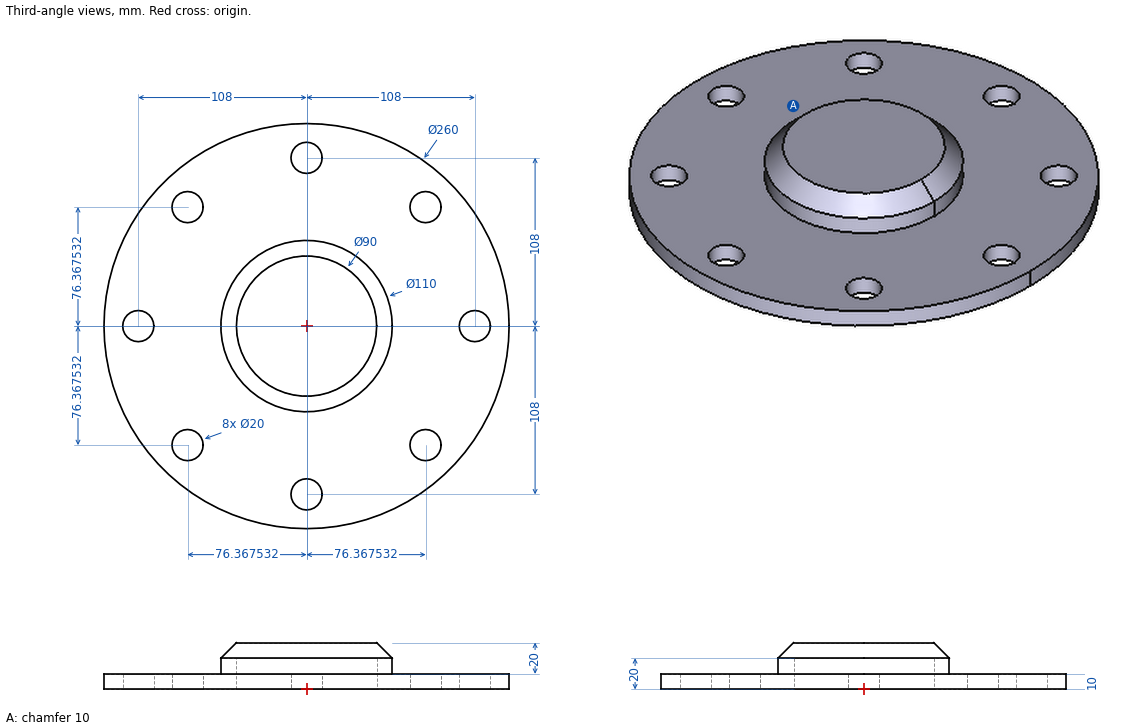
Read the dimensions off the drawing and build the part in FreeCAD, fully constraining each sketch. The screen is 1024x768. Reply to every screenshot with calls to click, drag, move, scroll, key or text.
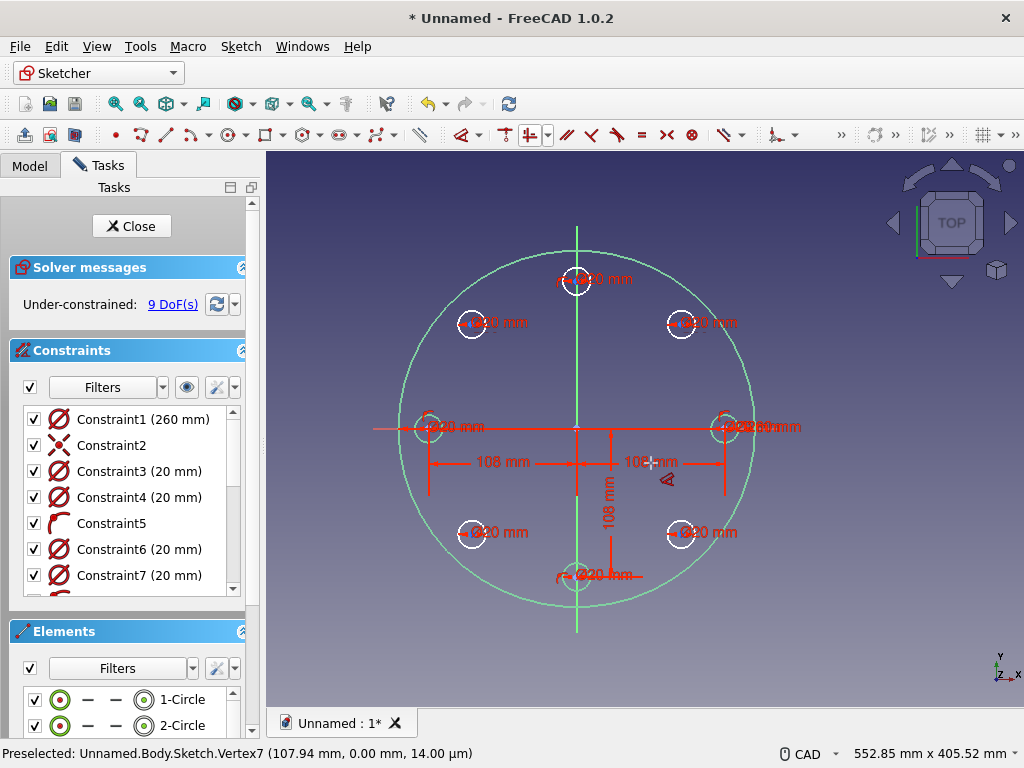
click(577, 281)
click(611, 355)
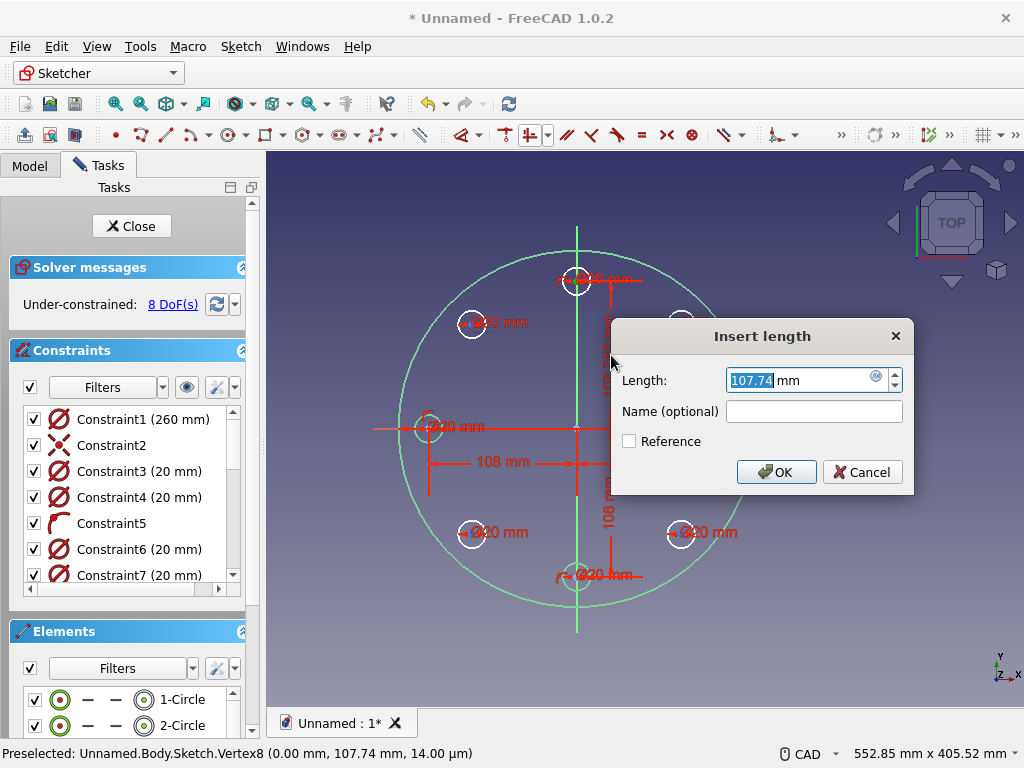
text(108)
key(Return)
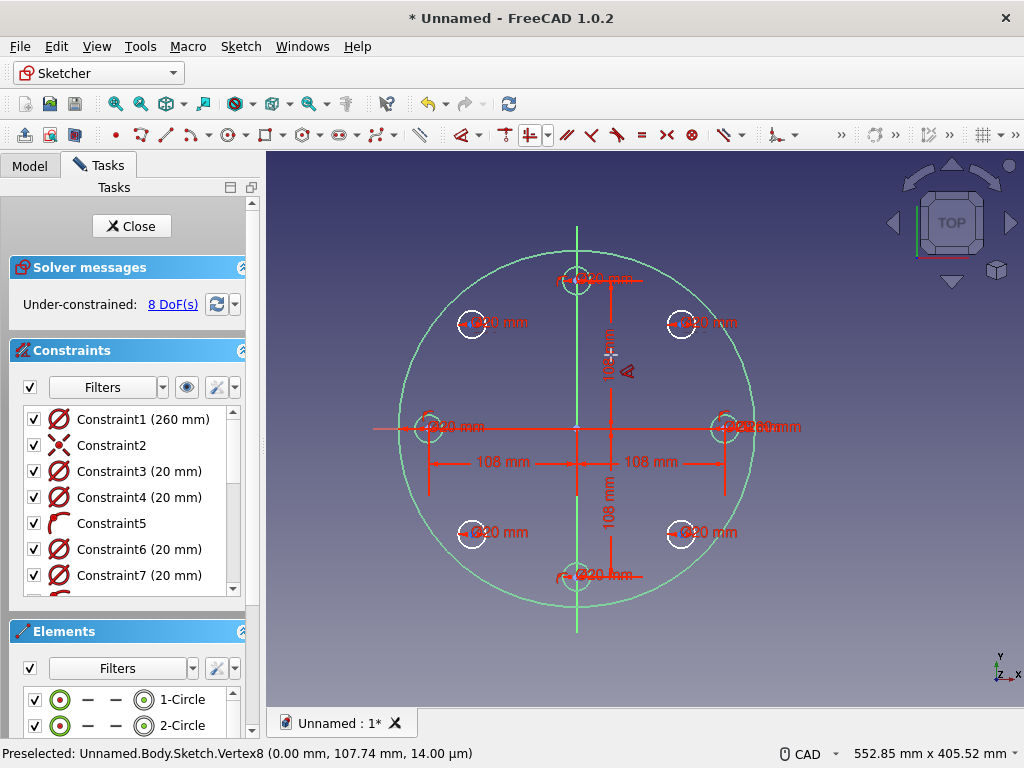
click(472, 534)
click(524, 568)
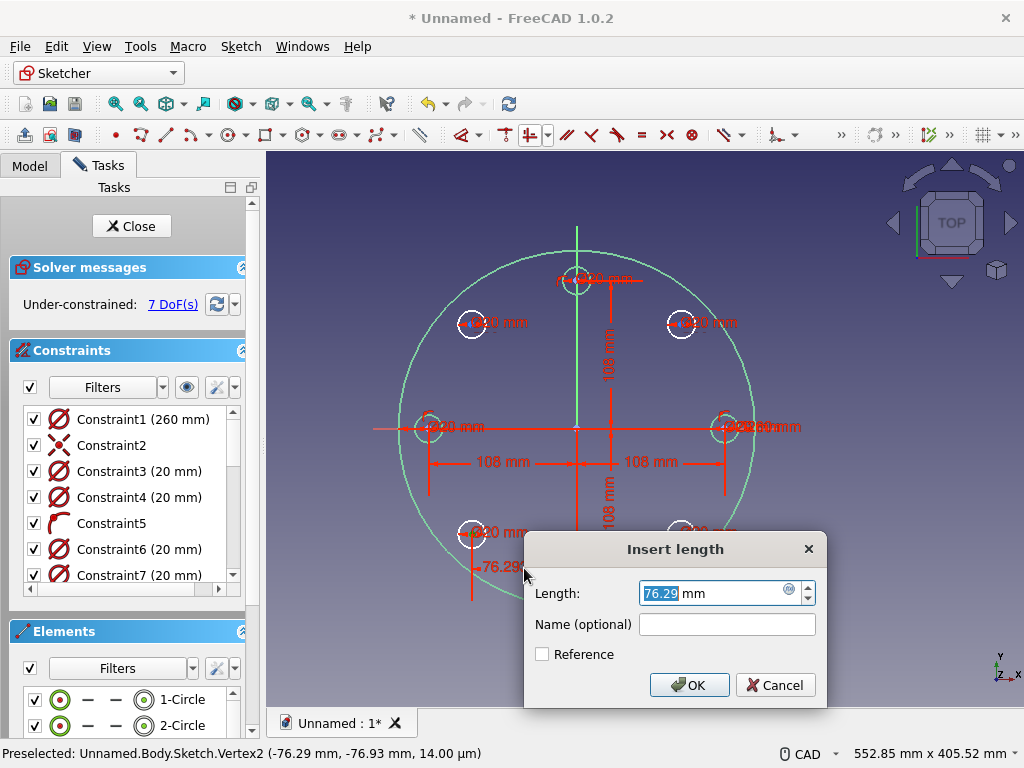
text(76.367532)
key(Return)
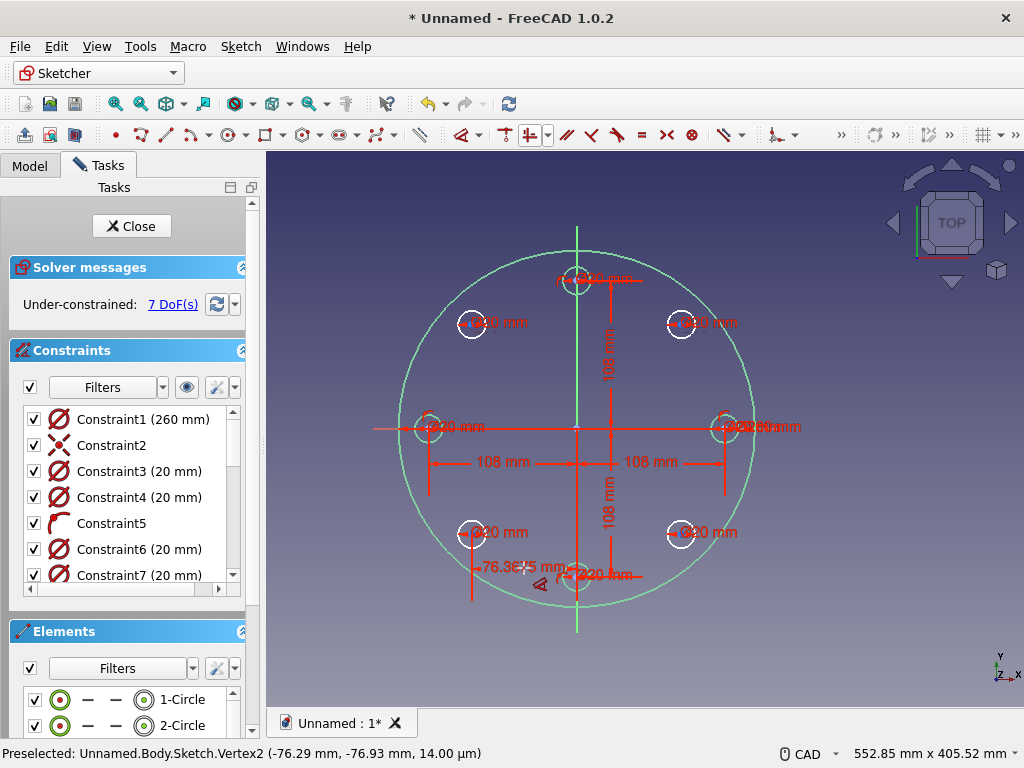
click(472, 534)
click(438, 506)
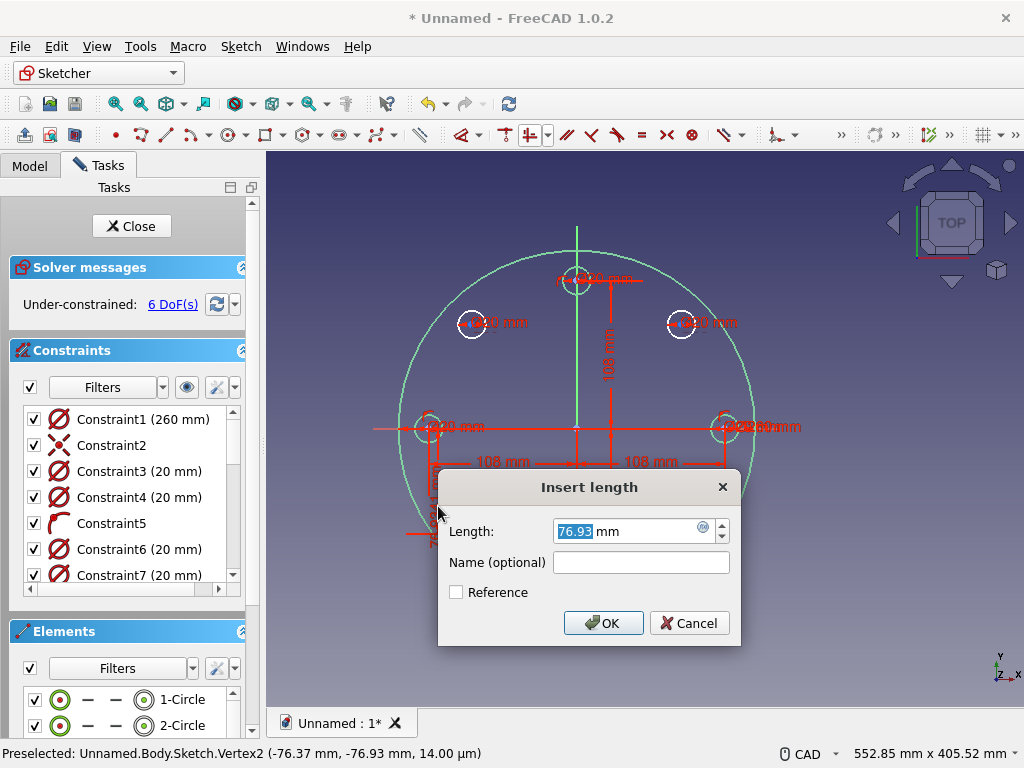
text(76.367532)
key(Return)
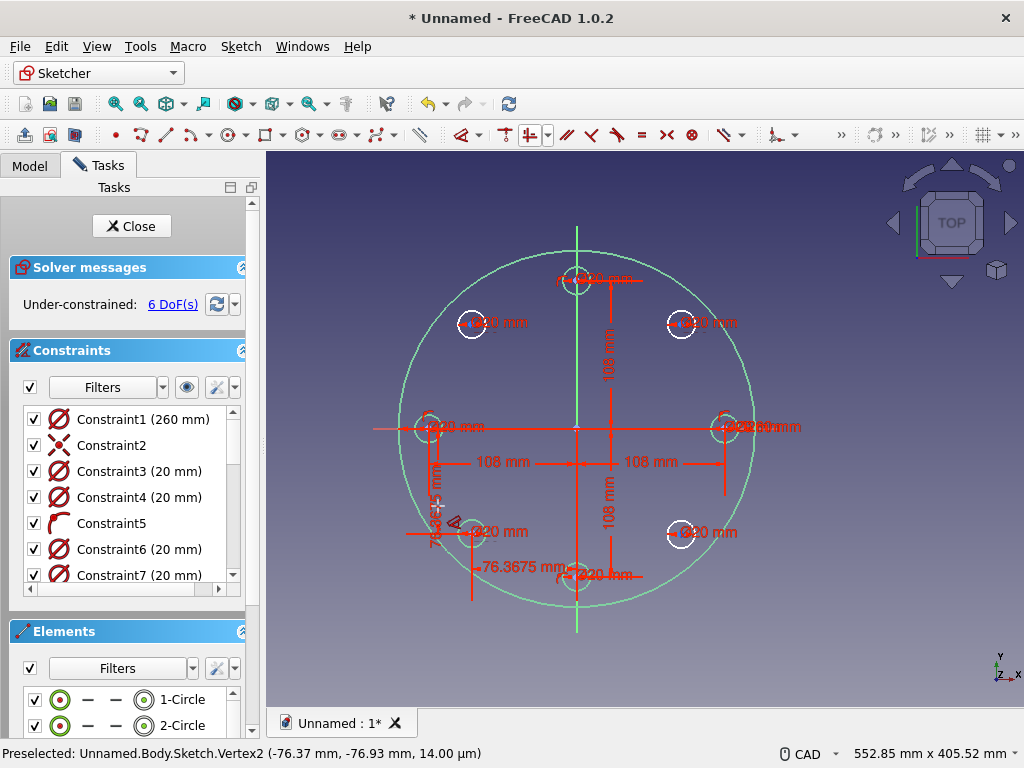
click(681, 534)
click(629, 568)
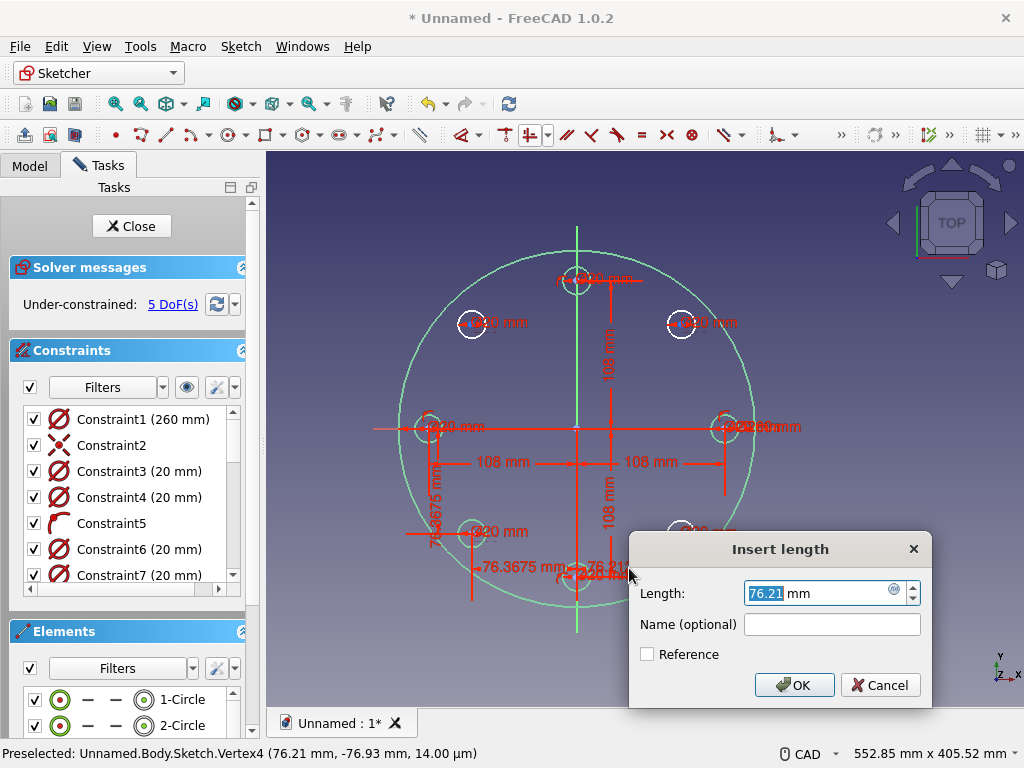
text(76.367532)
key(Return)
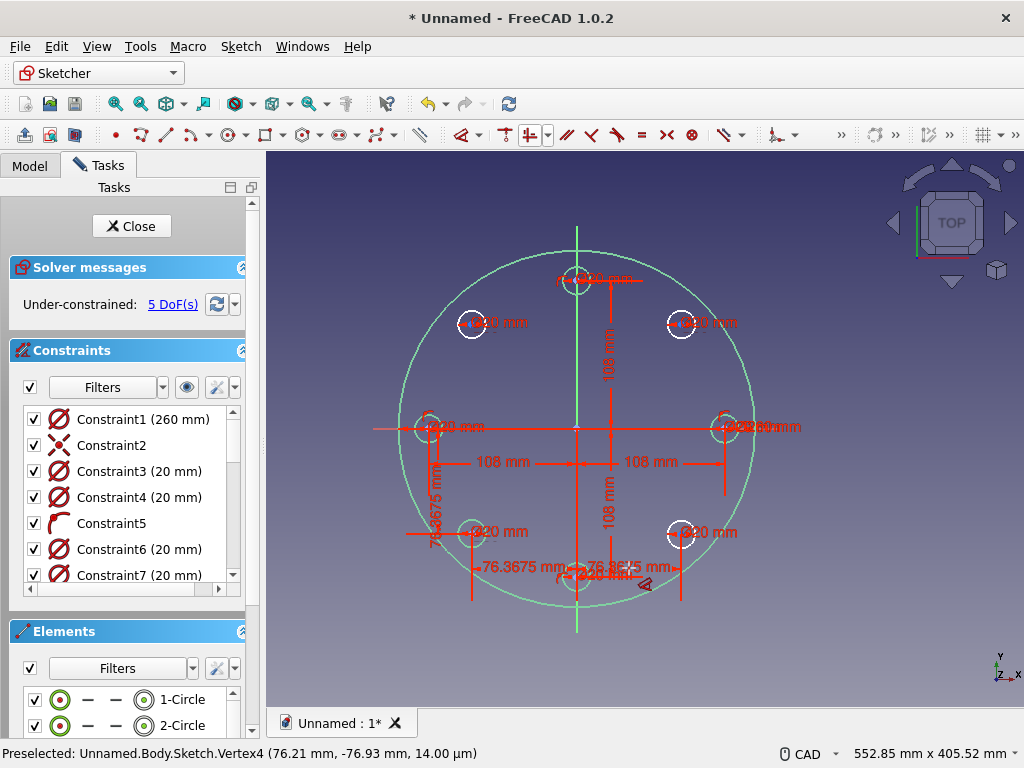
click(681, 534)
click(715, 506)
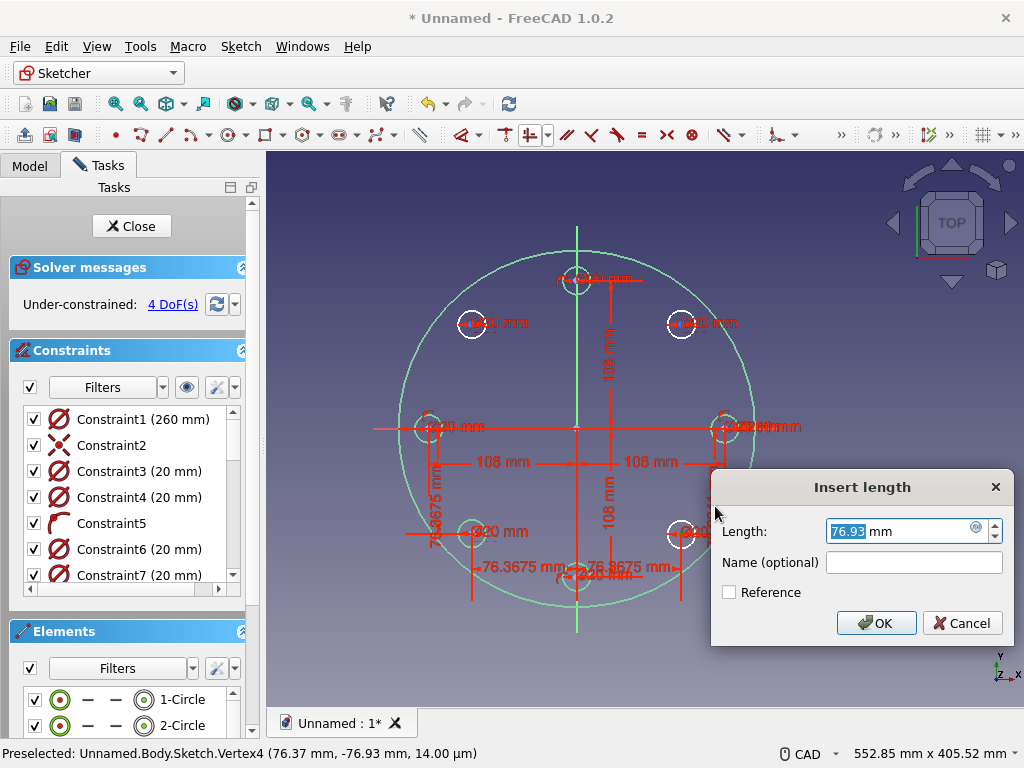
text(76.367532)
key(Return)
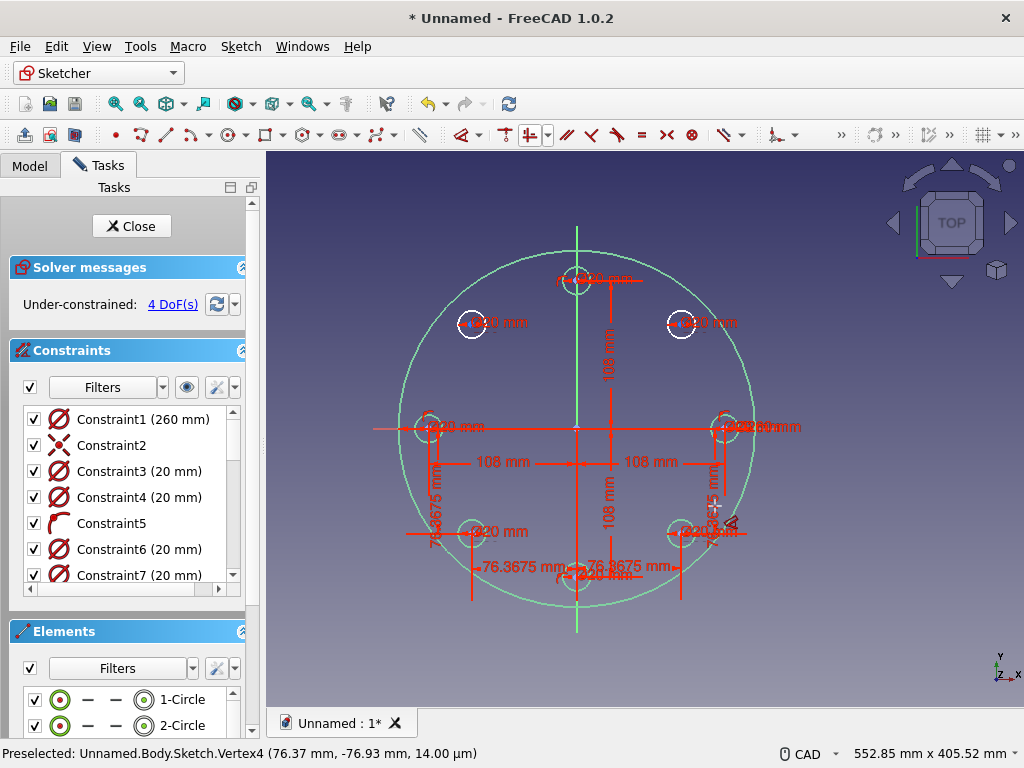
click(472, 324)
click(524, 290)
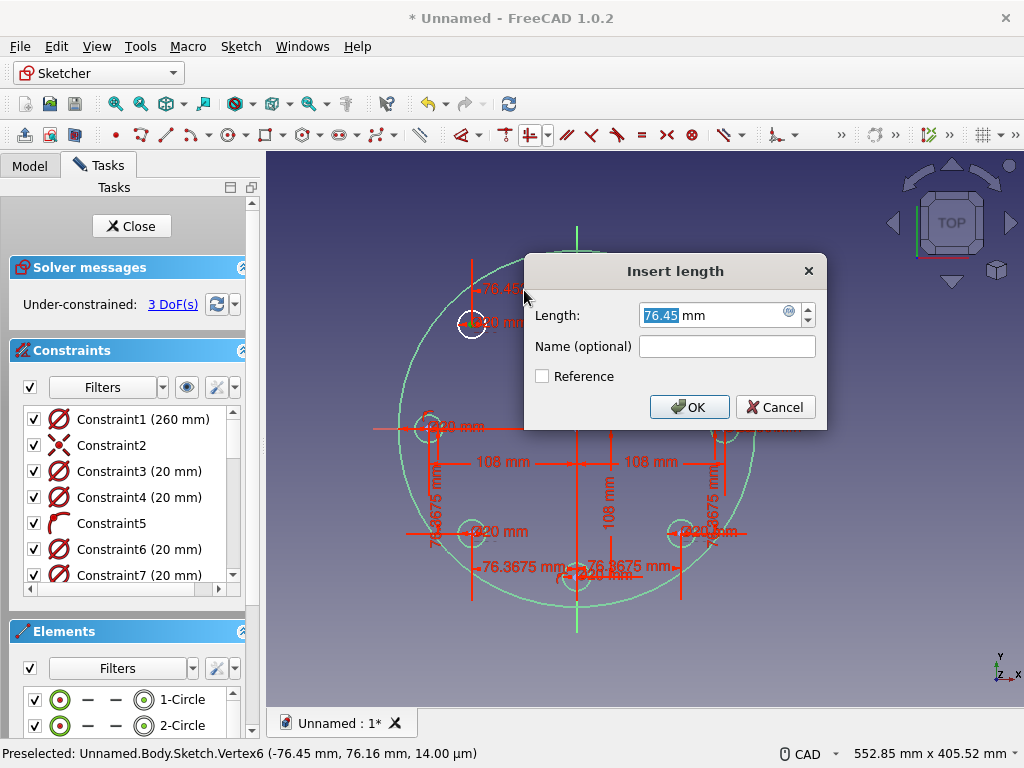
text(76.367532)
key(Return)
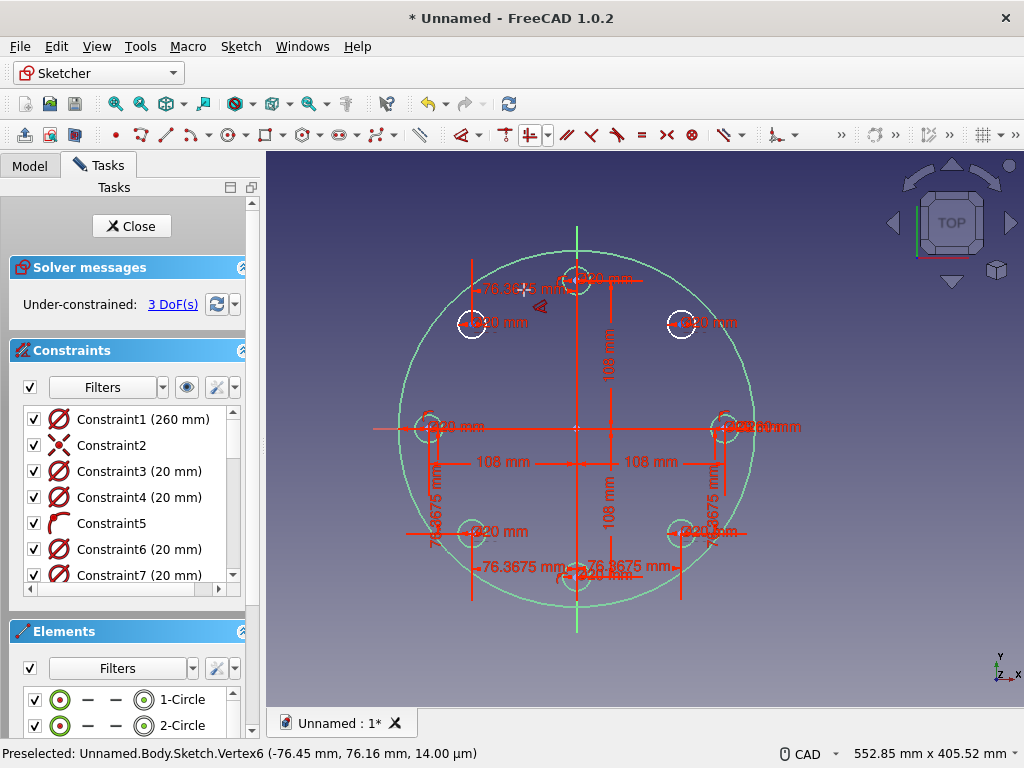
click(472, 324)
click(438, 377)